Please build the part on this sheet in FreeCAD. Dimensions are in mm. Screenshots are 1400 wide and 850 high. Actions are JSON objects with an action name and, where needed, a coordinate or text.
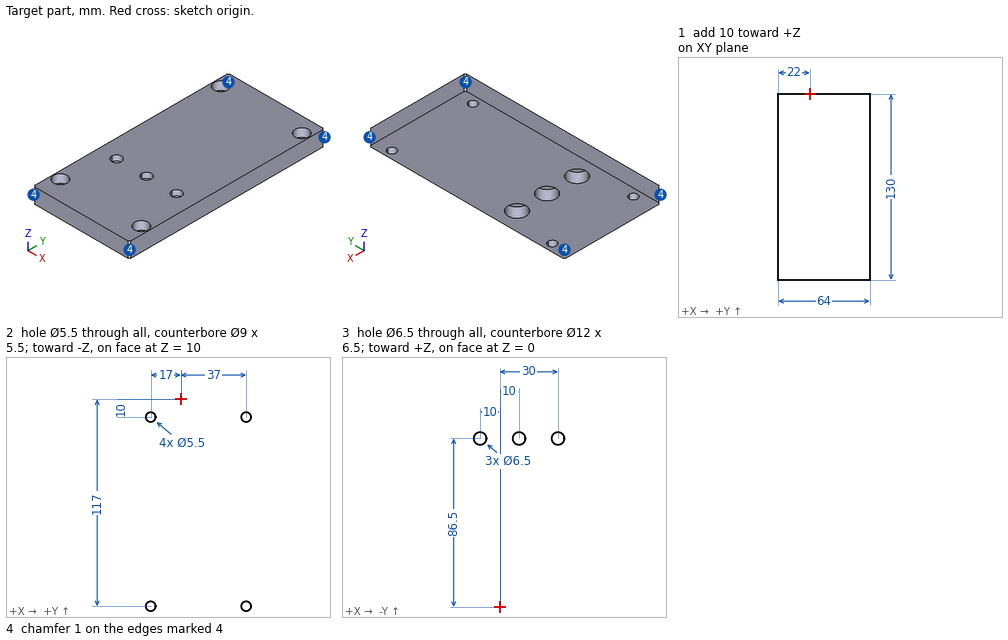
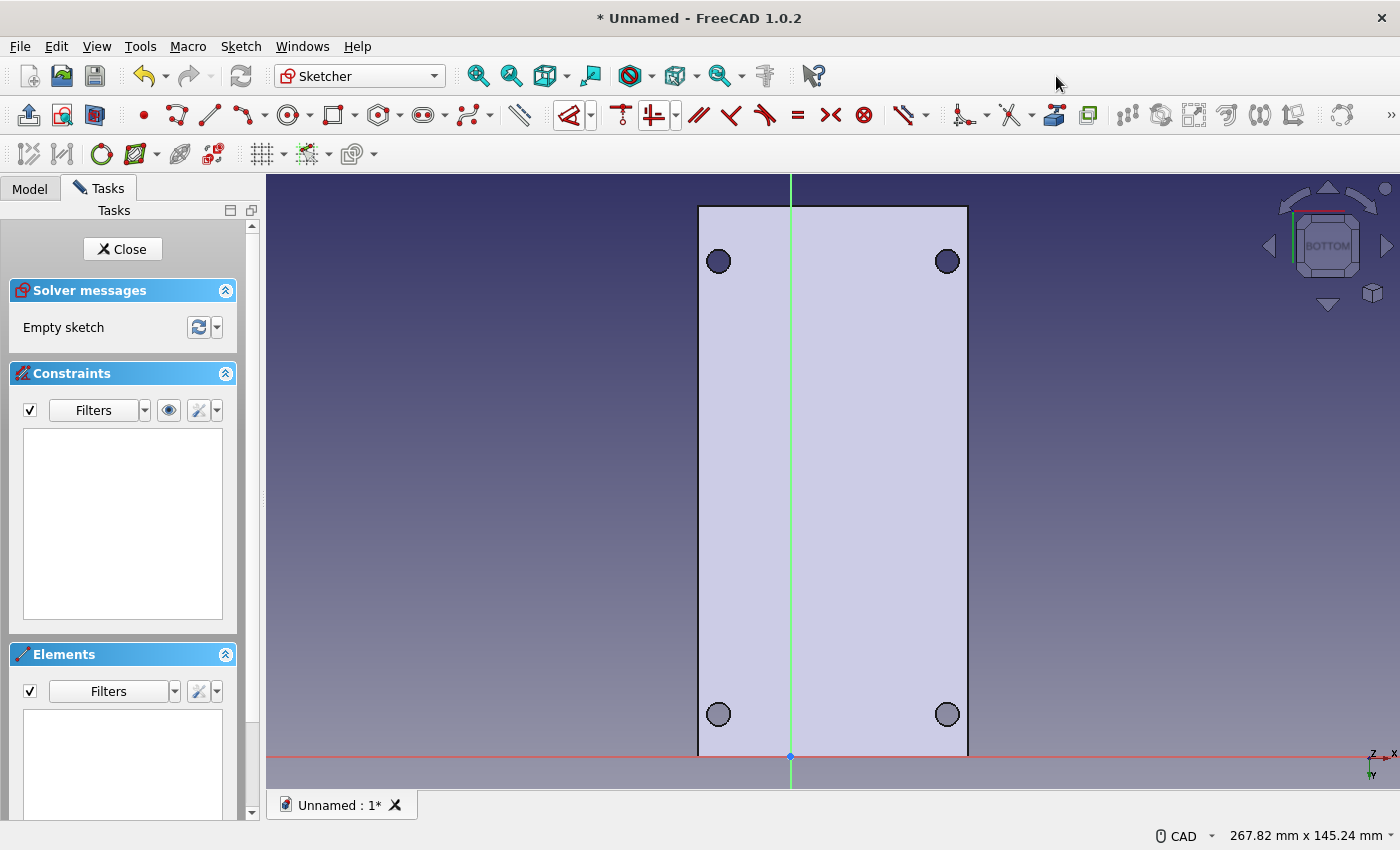
{"action": "scroll", "coordinate": [455, 202], "scroll_direction": "down", "scroll_amount": 1}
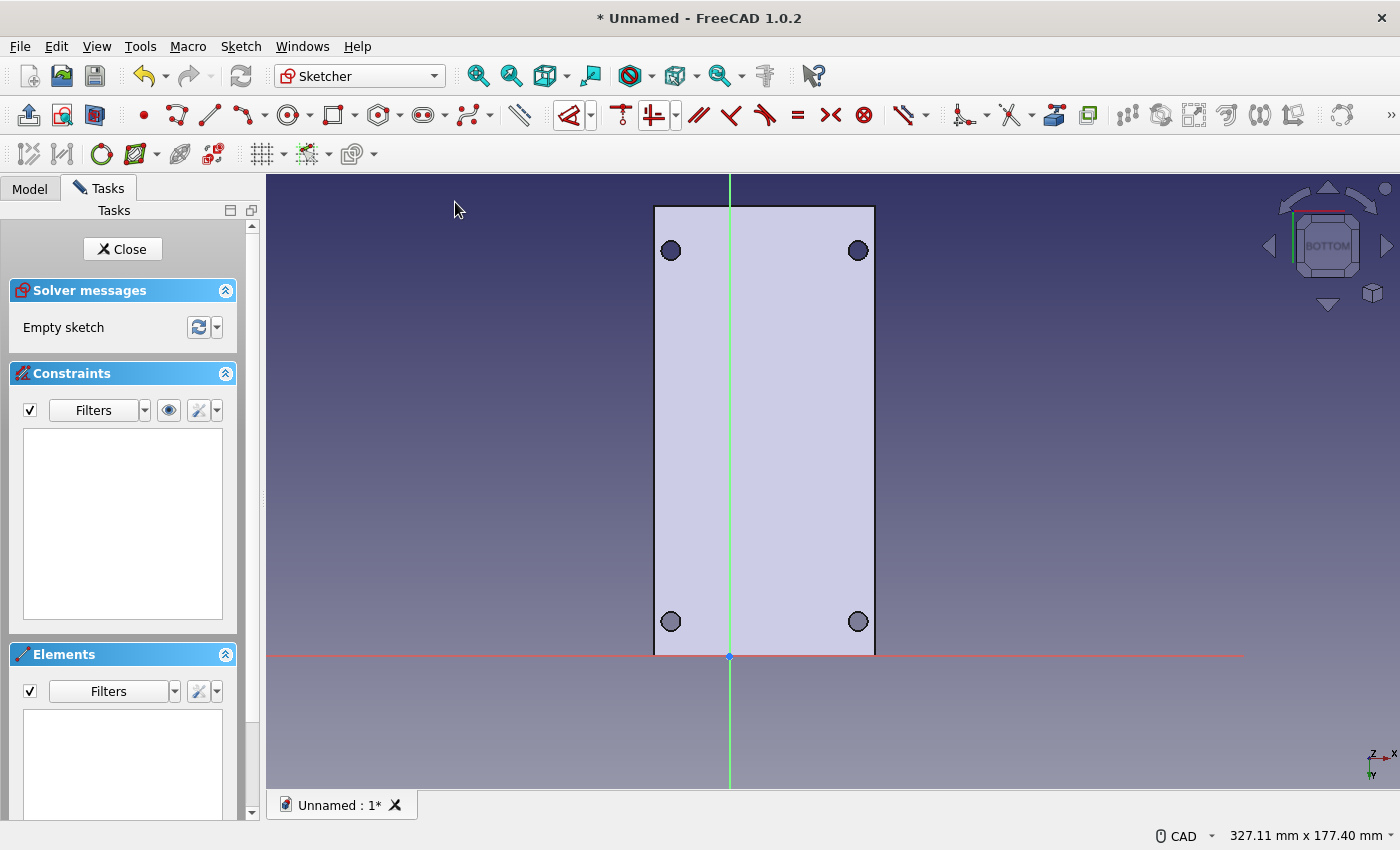
{"action": "key", "text": "g c"}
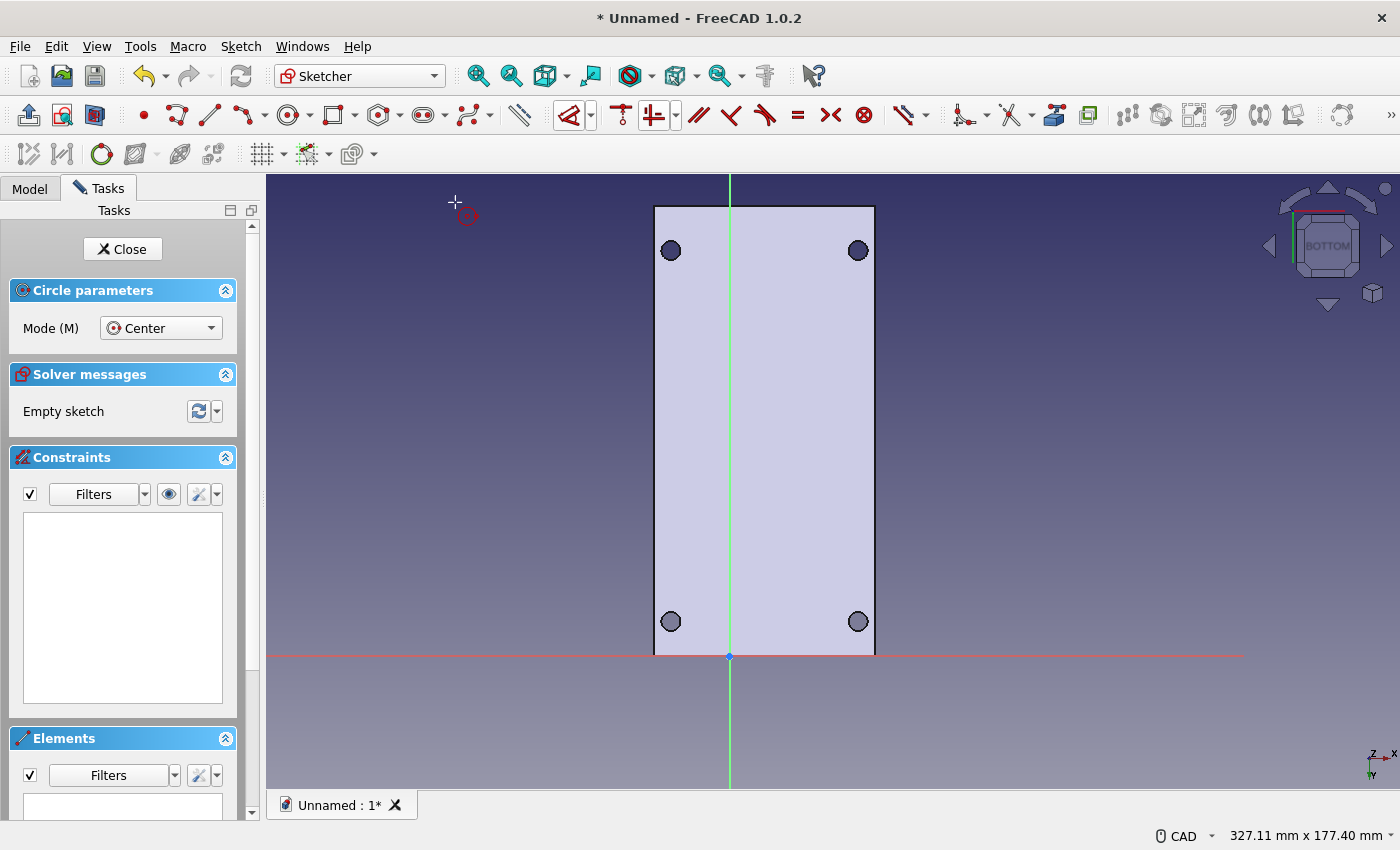
{"action": "scroll", "coordinate": [695, 356], "scroll_direction": "up", "scroll_amount": 4}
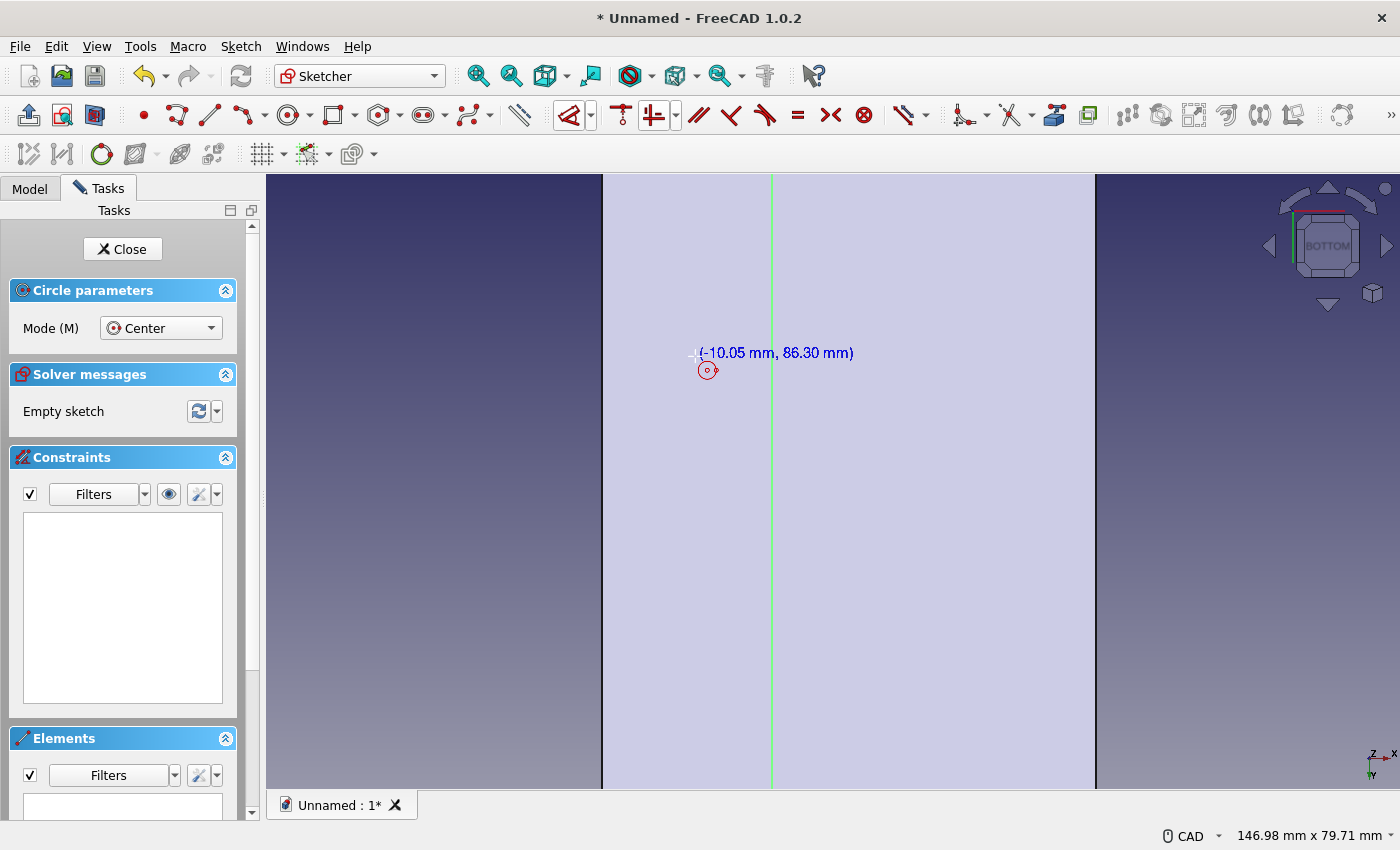
{"action": "left_click", "coordinate": [695, 356]}
{"action": "mouse_move", "coordinate": [713, 339]}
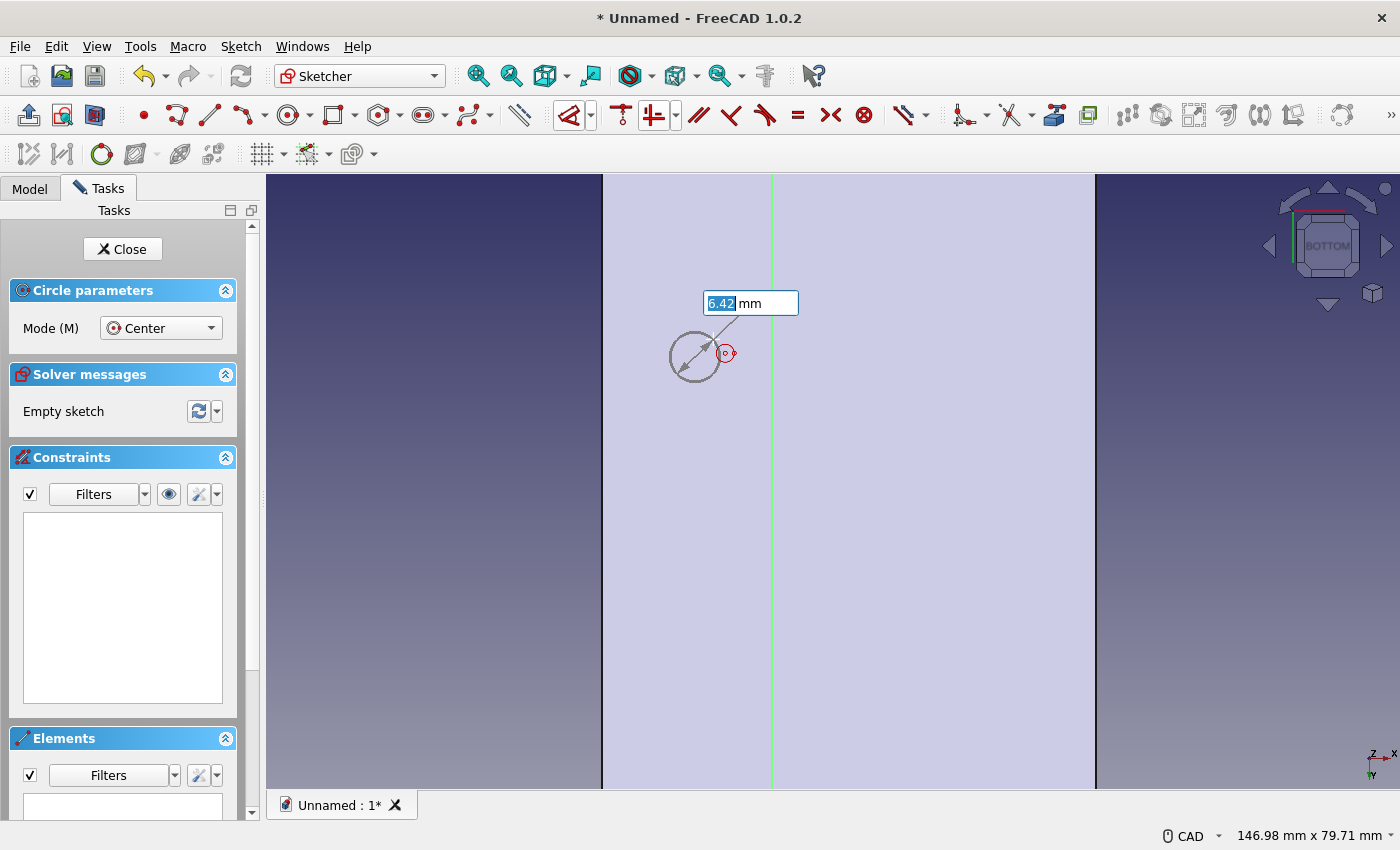
{"action": "type", "text": "6.5"}
{"action": "key", "text": "Return"}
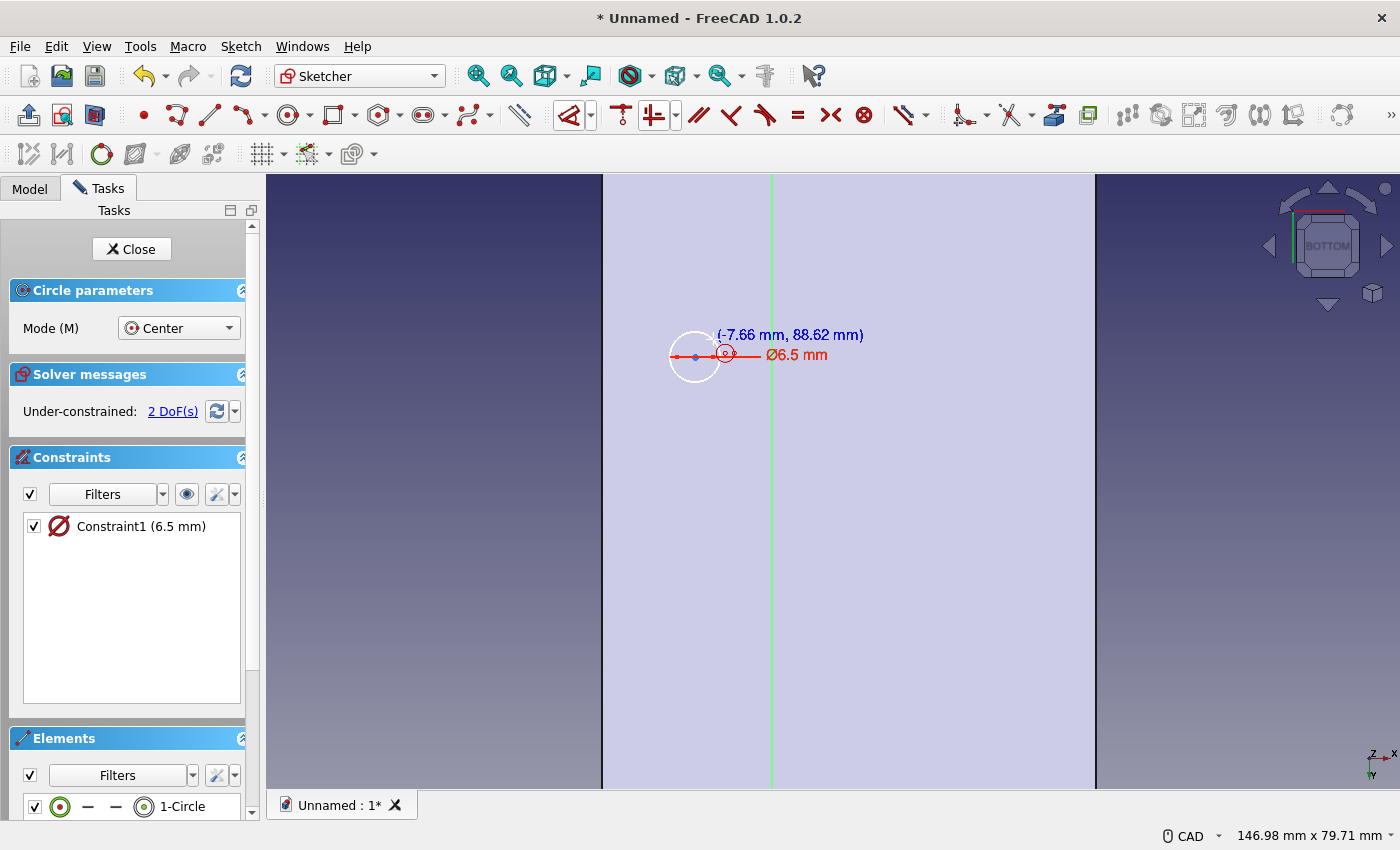
{"action": "left_click", "coordinate": [849, 356]}
{"action": "mouse_move", "coordinate": [867, 339]}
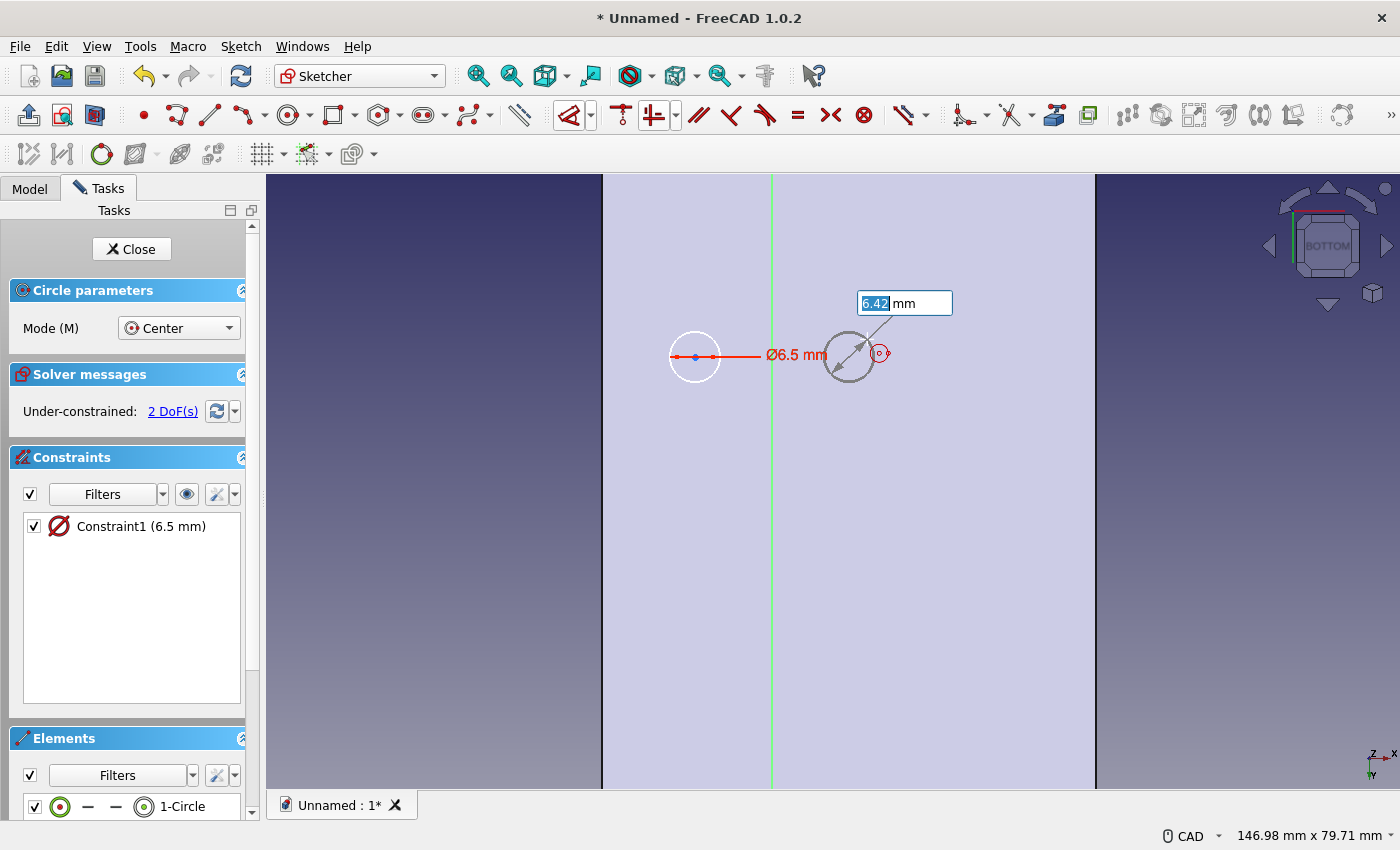
{"action": "type", "text": "6.5"}
{"action": "key", "text": "Return"}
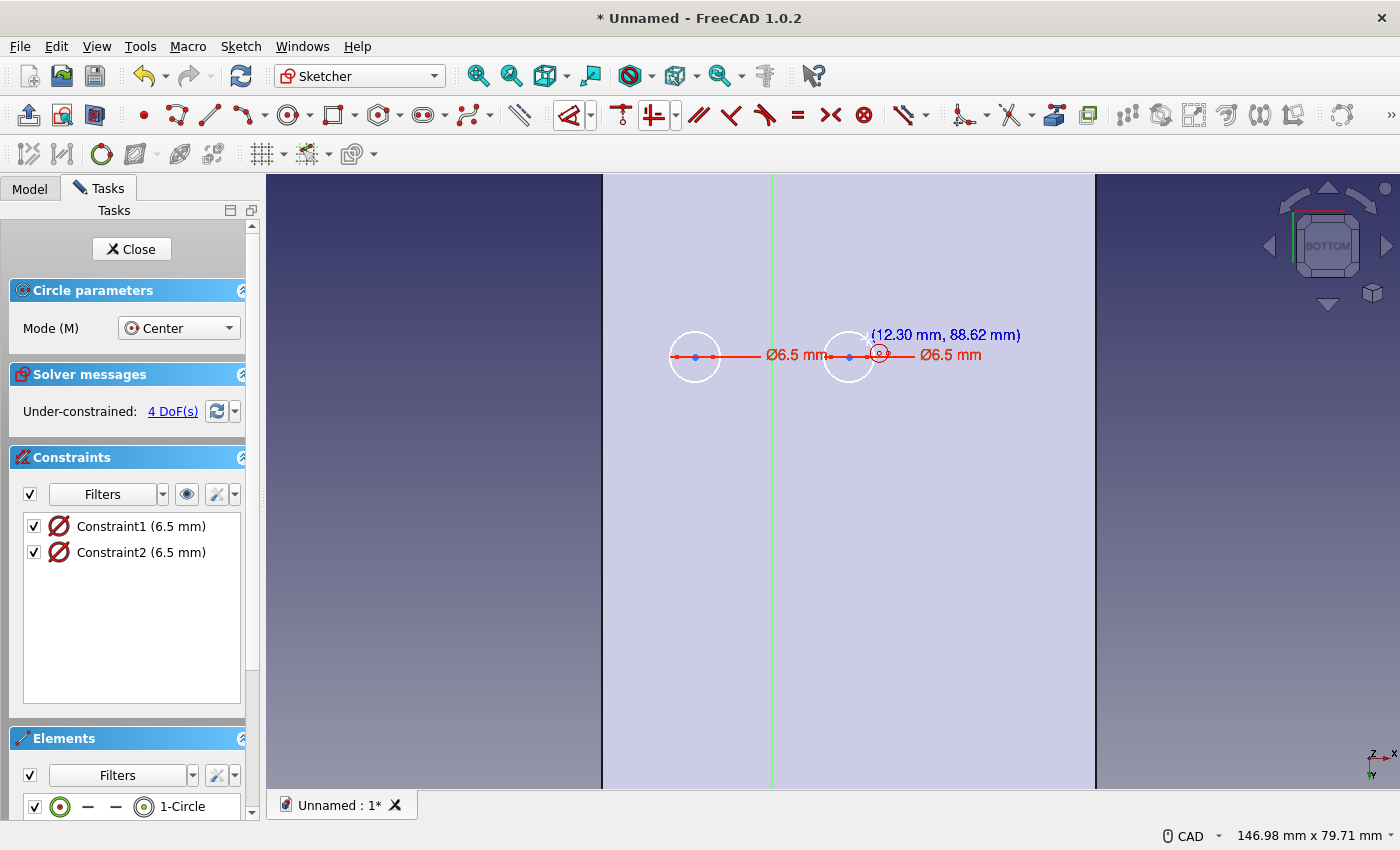
{"action": "left_click", "coordinate": [1004, 356]}
{"action": "mouse_move", "coordinate": [1021, 339]}